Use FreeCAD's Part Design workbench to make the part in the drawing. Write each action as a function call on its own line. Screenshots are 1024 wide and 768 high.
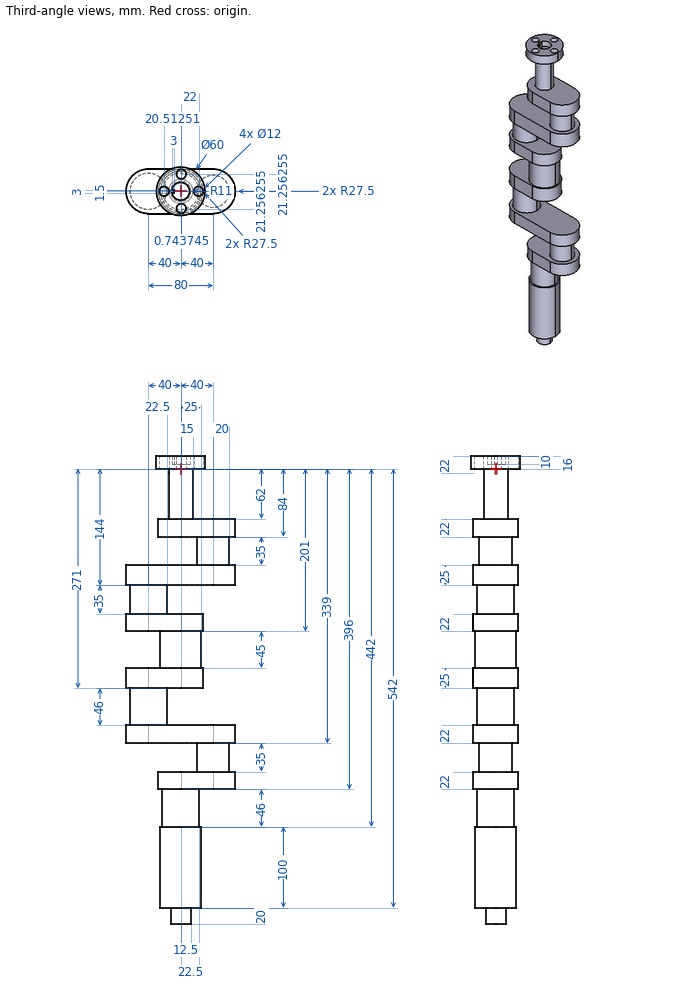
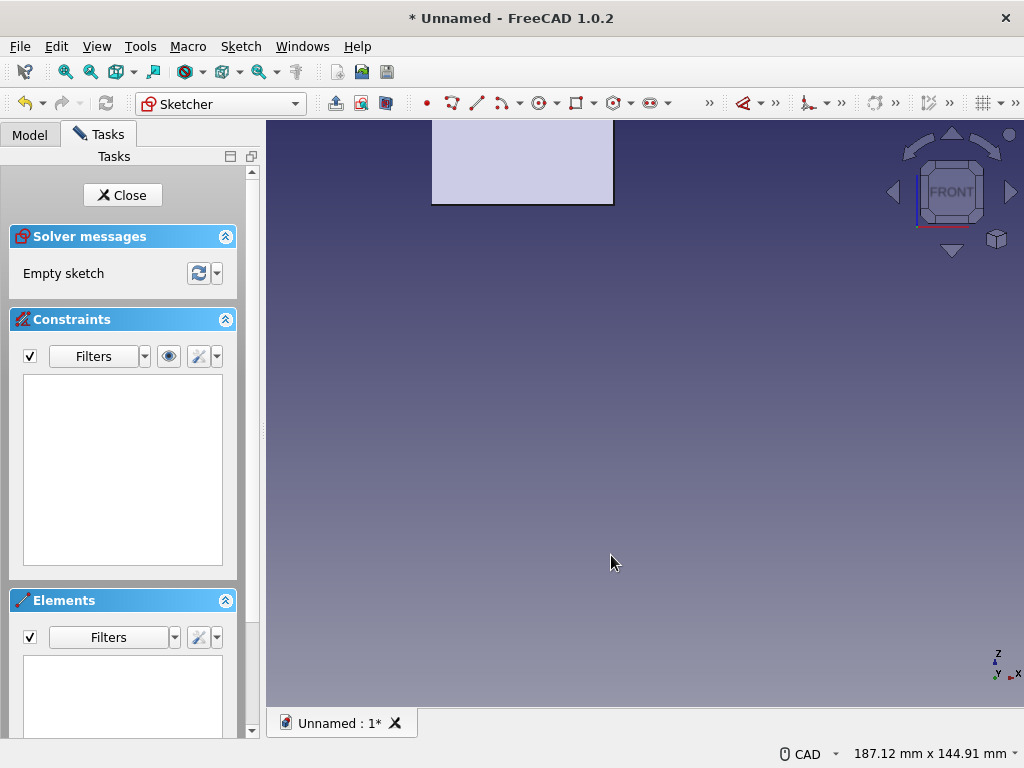
key(g)
key(r)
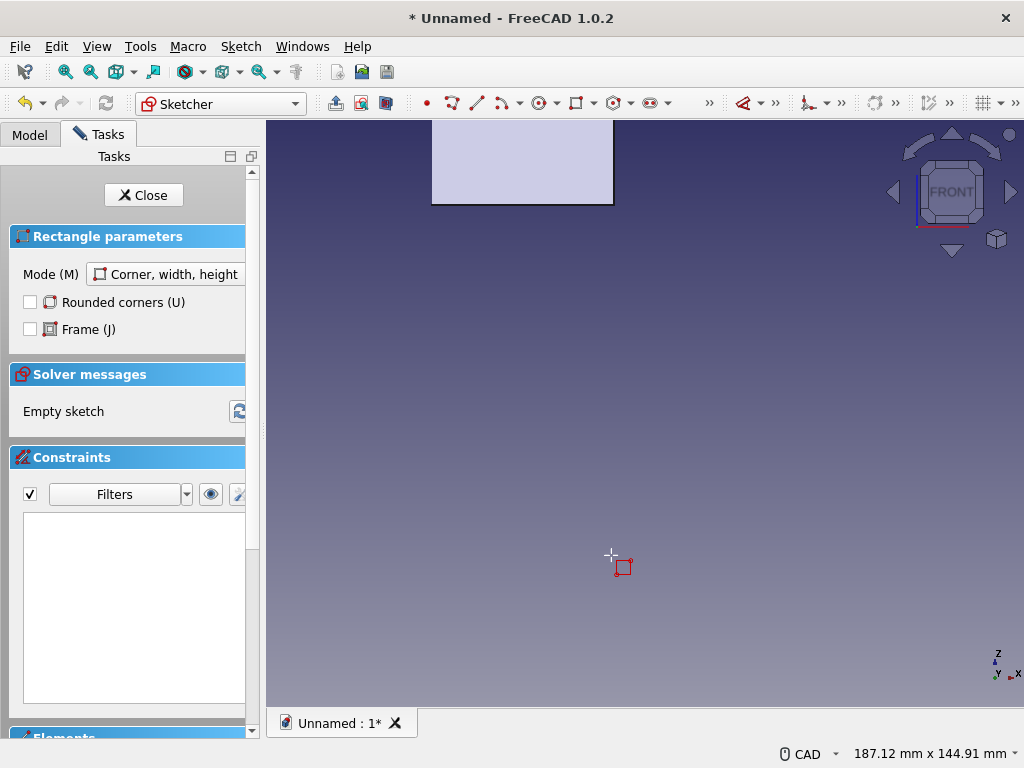
click(523, 205)
move(624, 610)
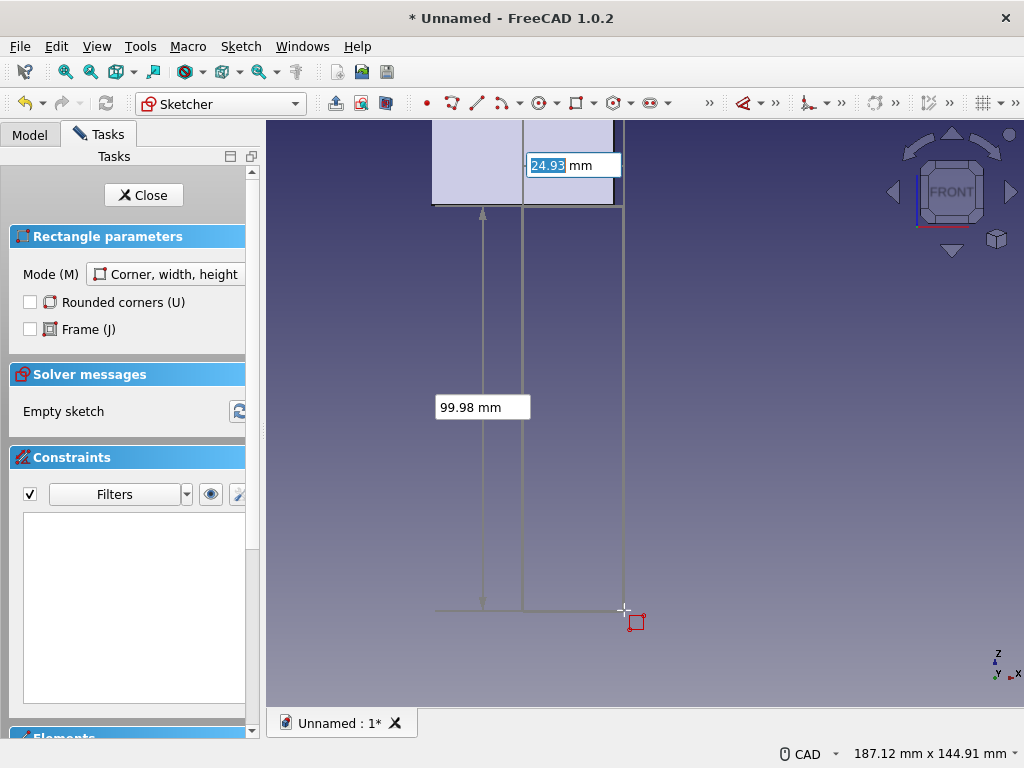
text(25)
key(Tab)
text(100)
key(Return)
key(Escape)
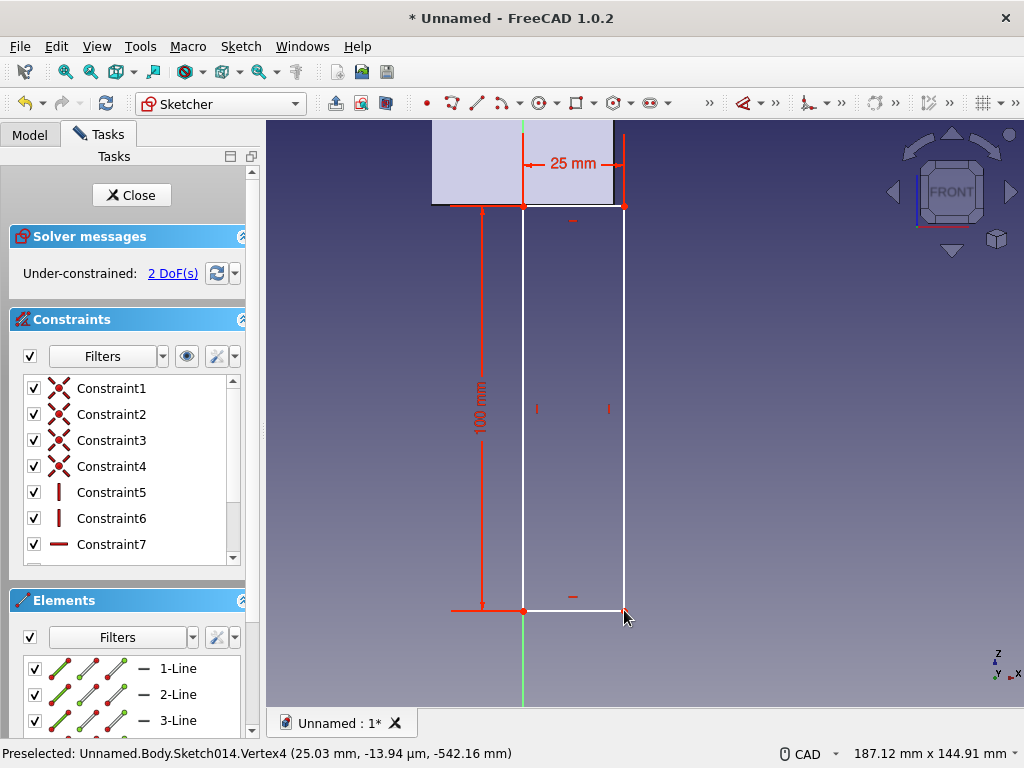
click(523, 206)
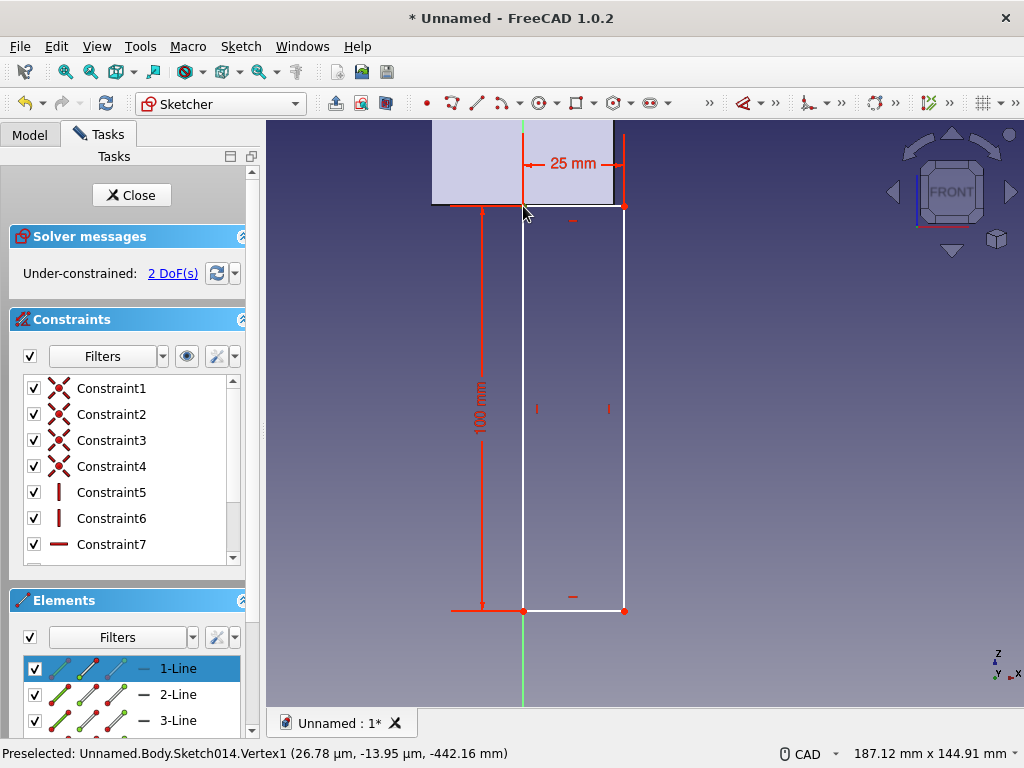
click(523, 641)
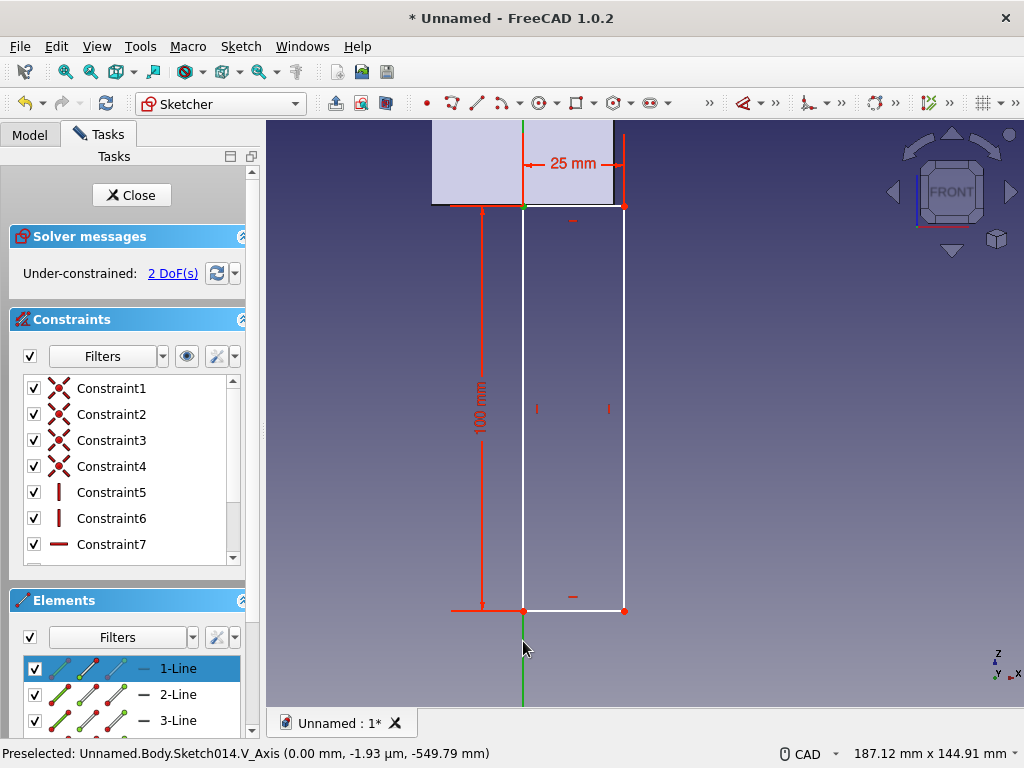
key(c)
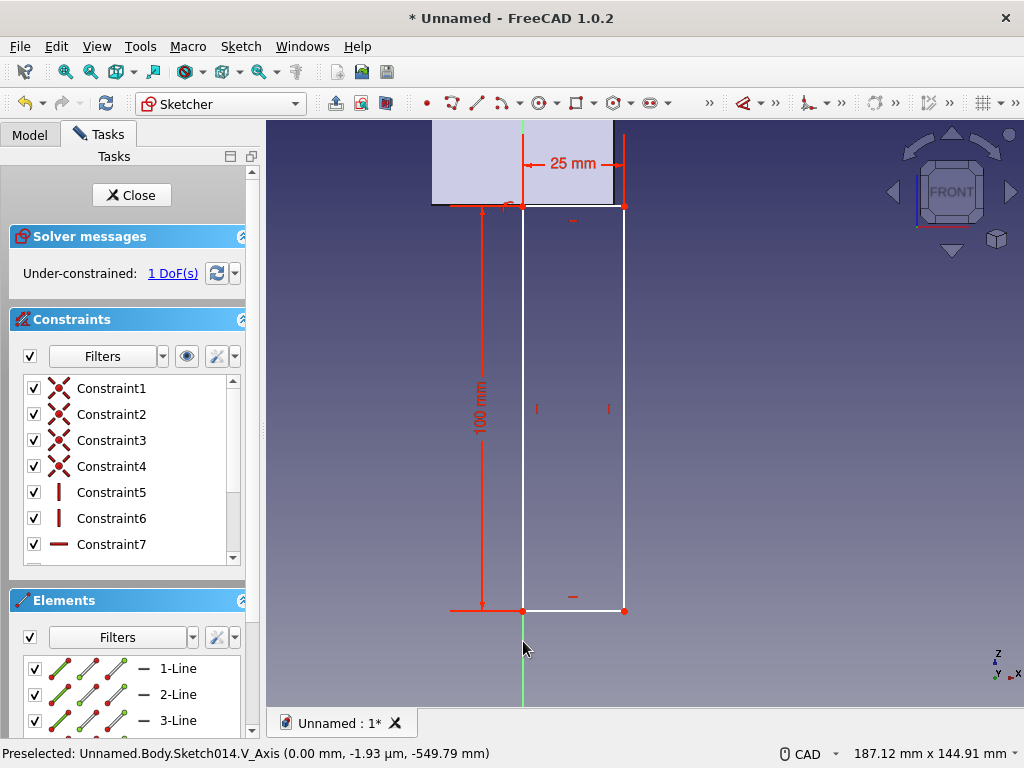
click(742, 104)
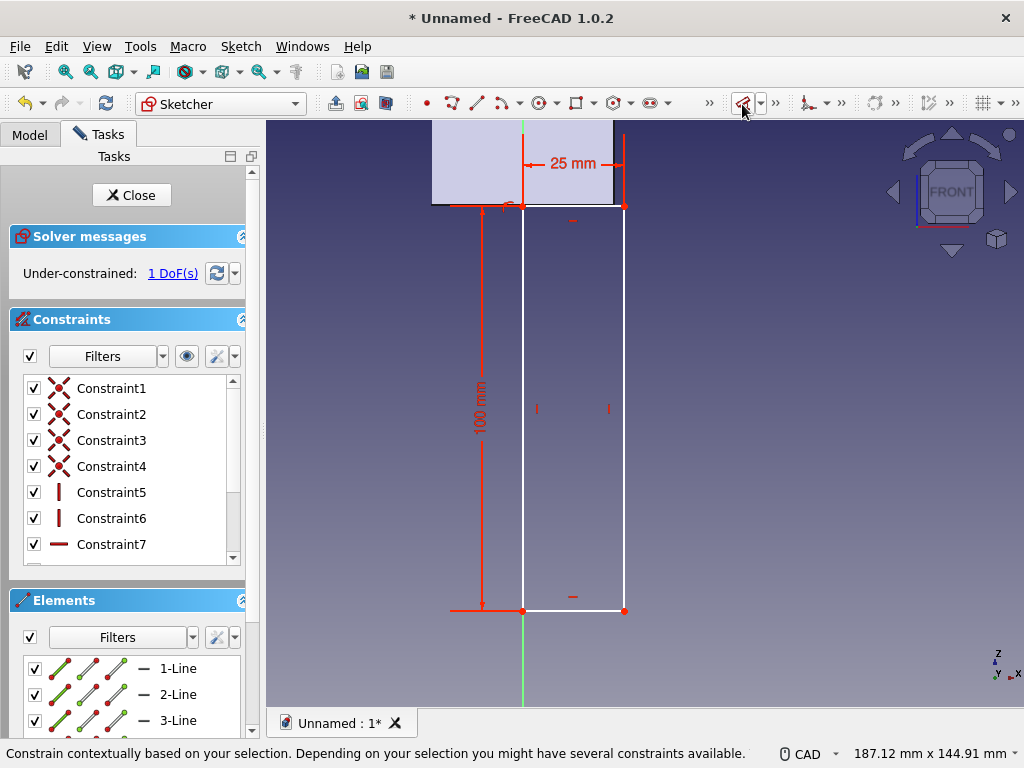
click(523, 206)
click(489, 177)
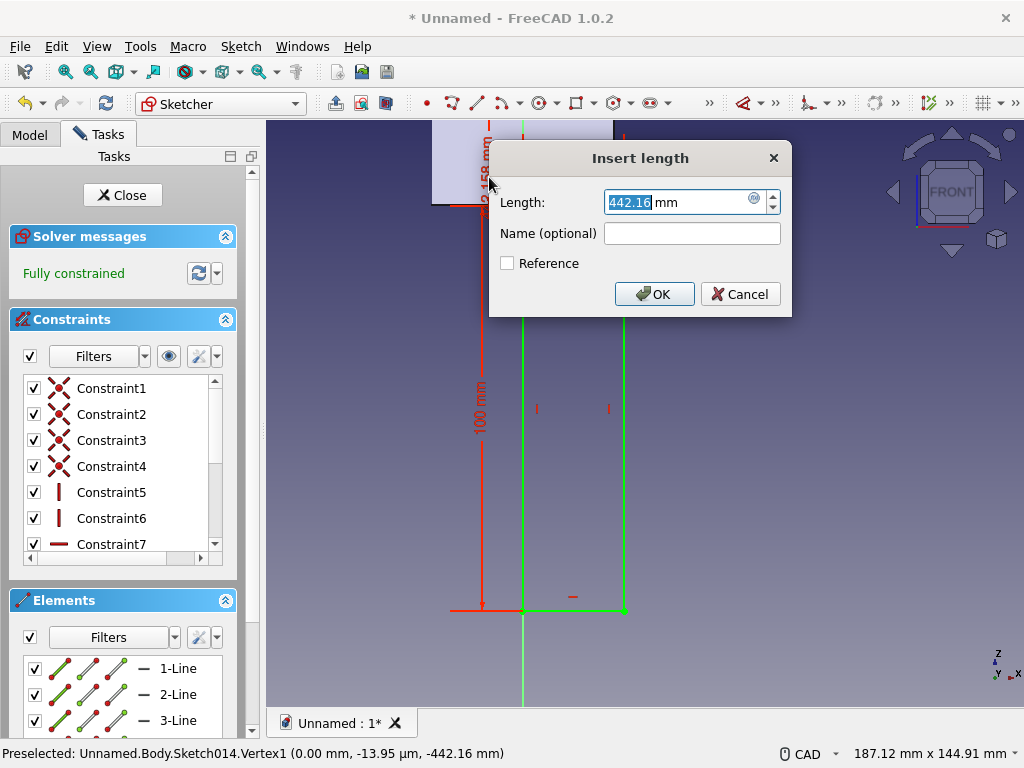
text(442)
key(Return)
key(Escape)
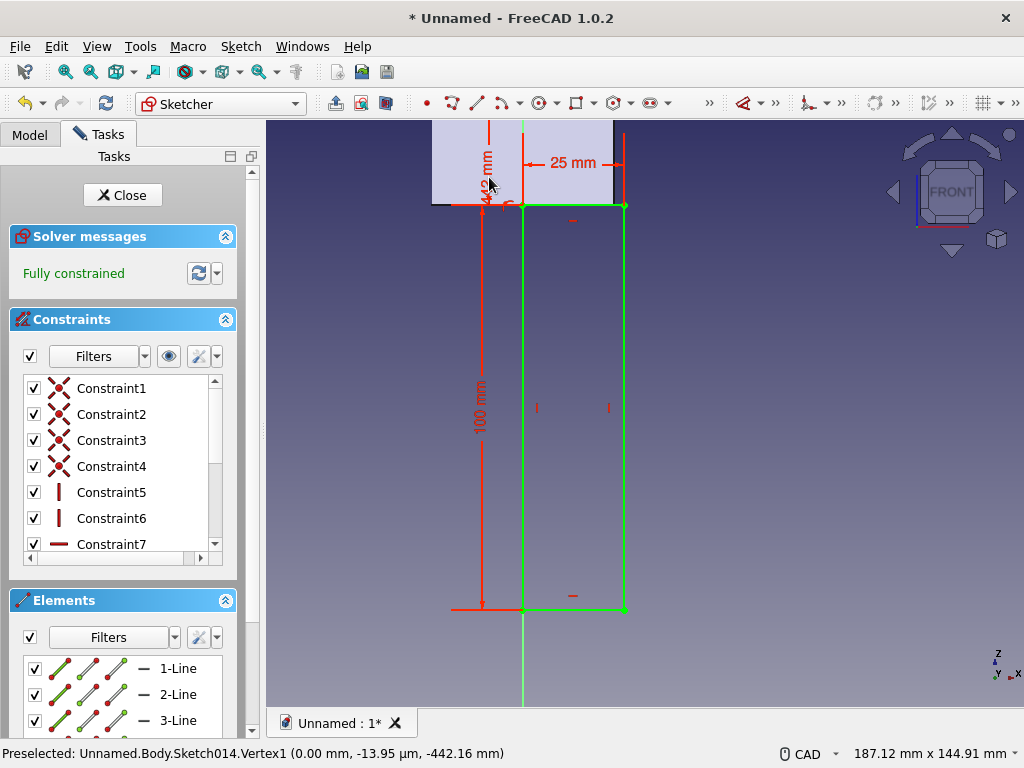
click(123, 195)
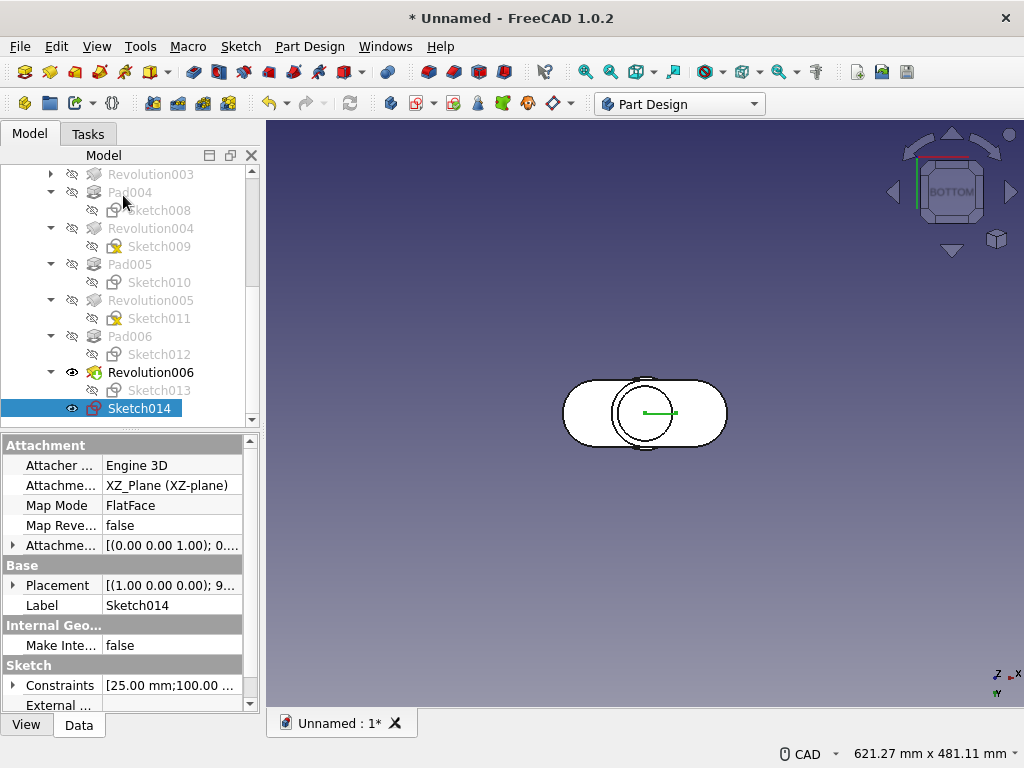
click(50, 72)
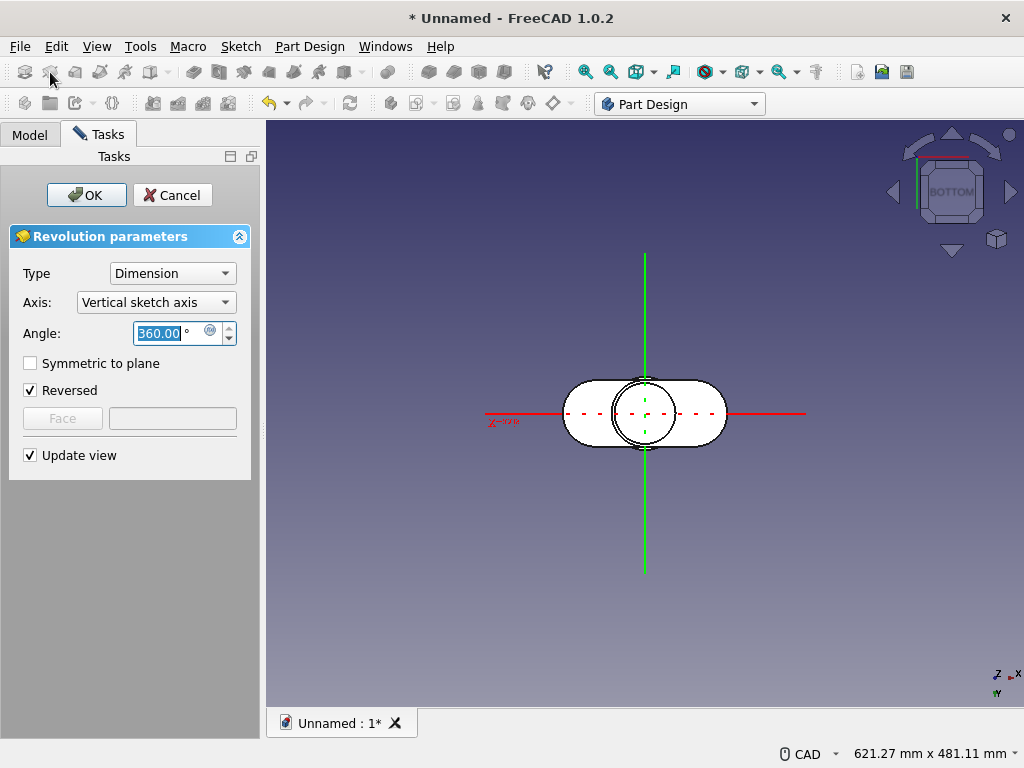
click(87, 195)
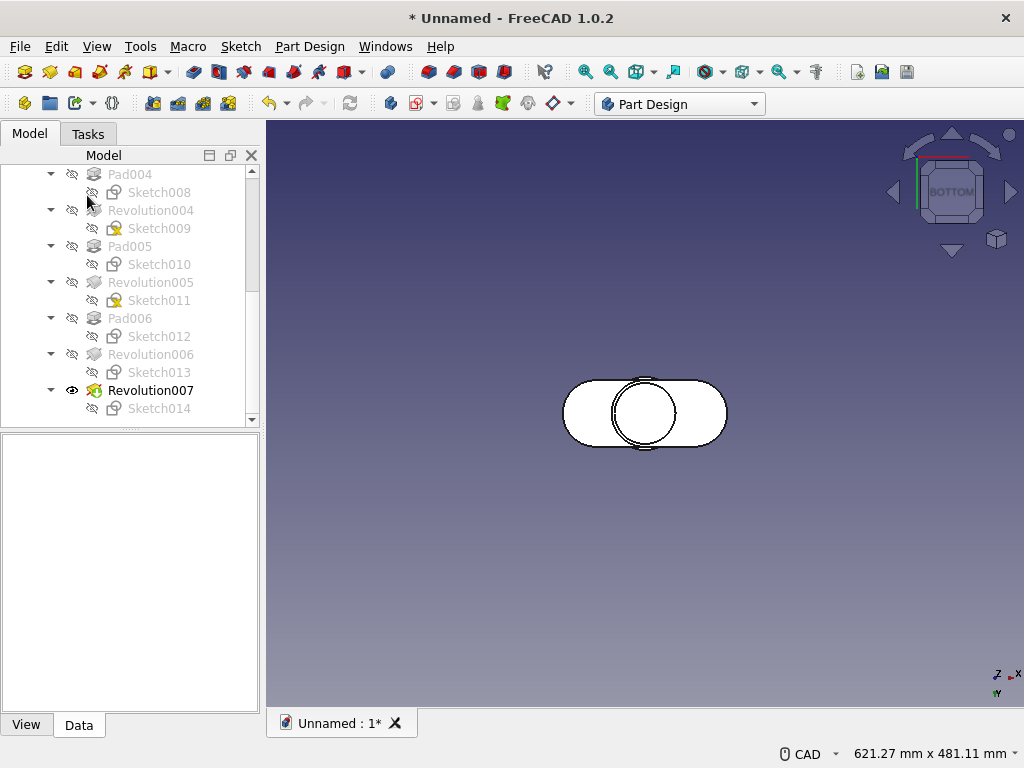
key(v)
key(f)